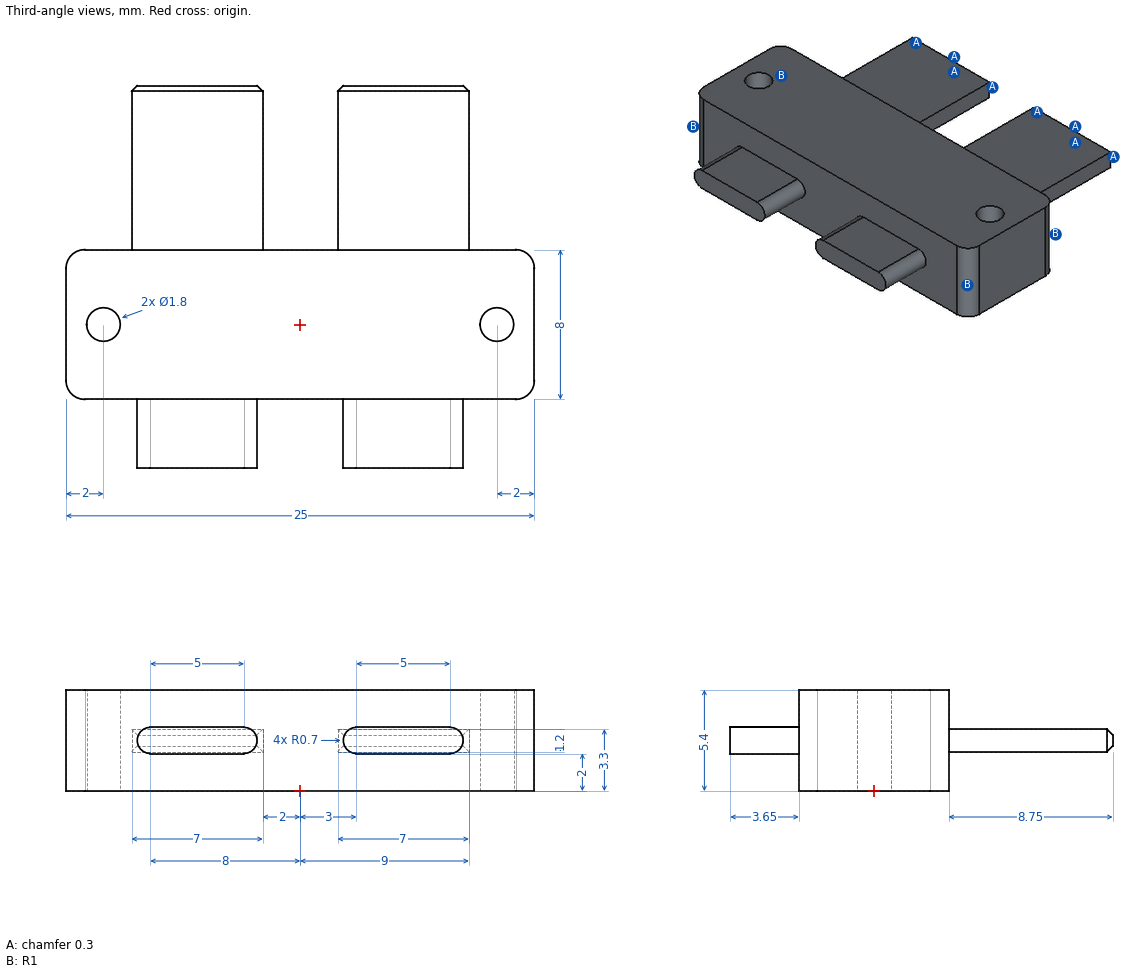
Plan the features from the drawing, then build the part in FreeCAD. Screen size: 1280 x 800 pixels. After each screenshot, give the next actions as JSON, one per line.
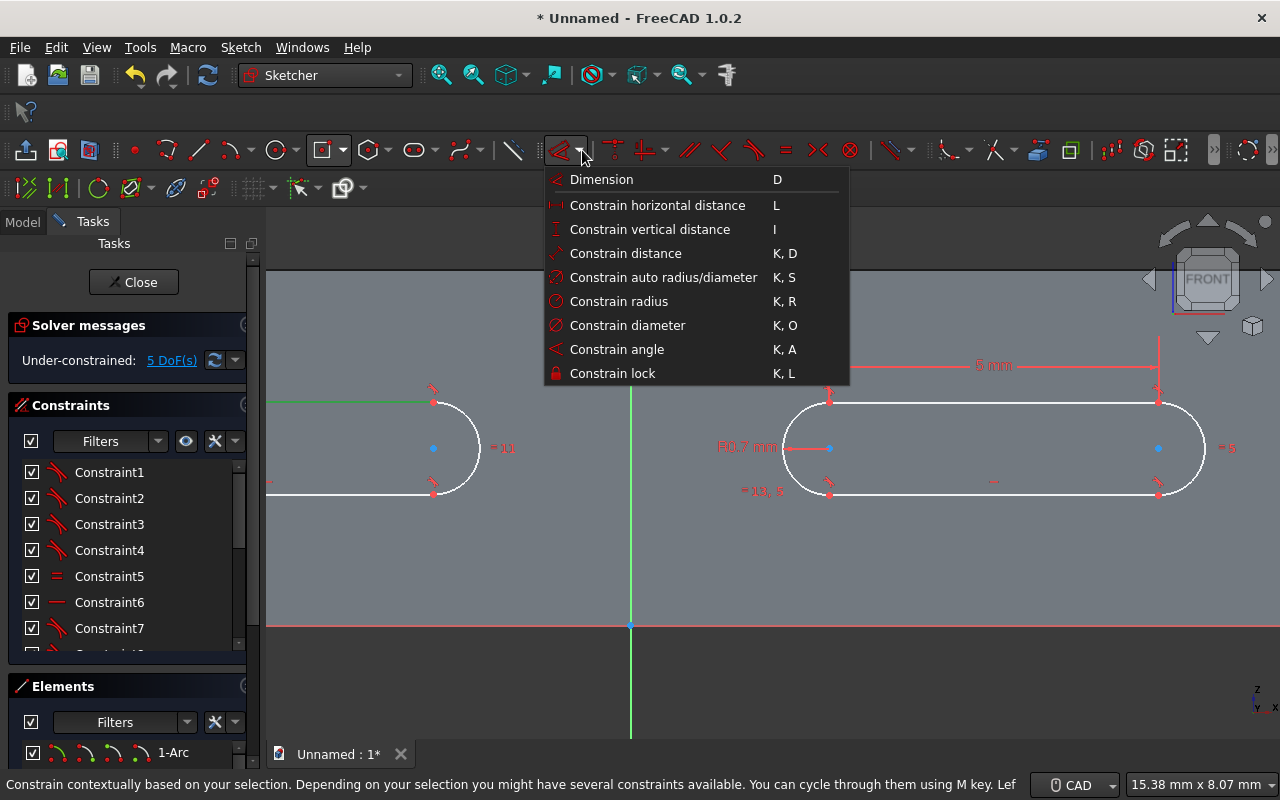
{"action": "left_click", "coordinate": [697, 205]}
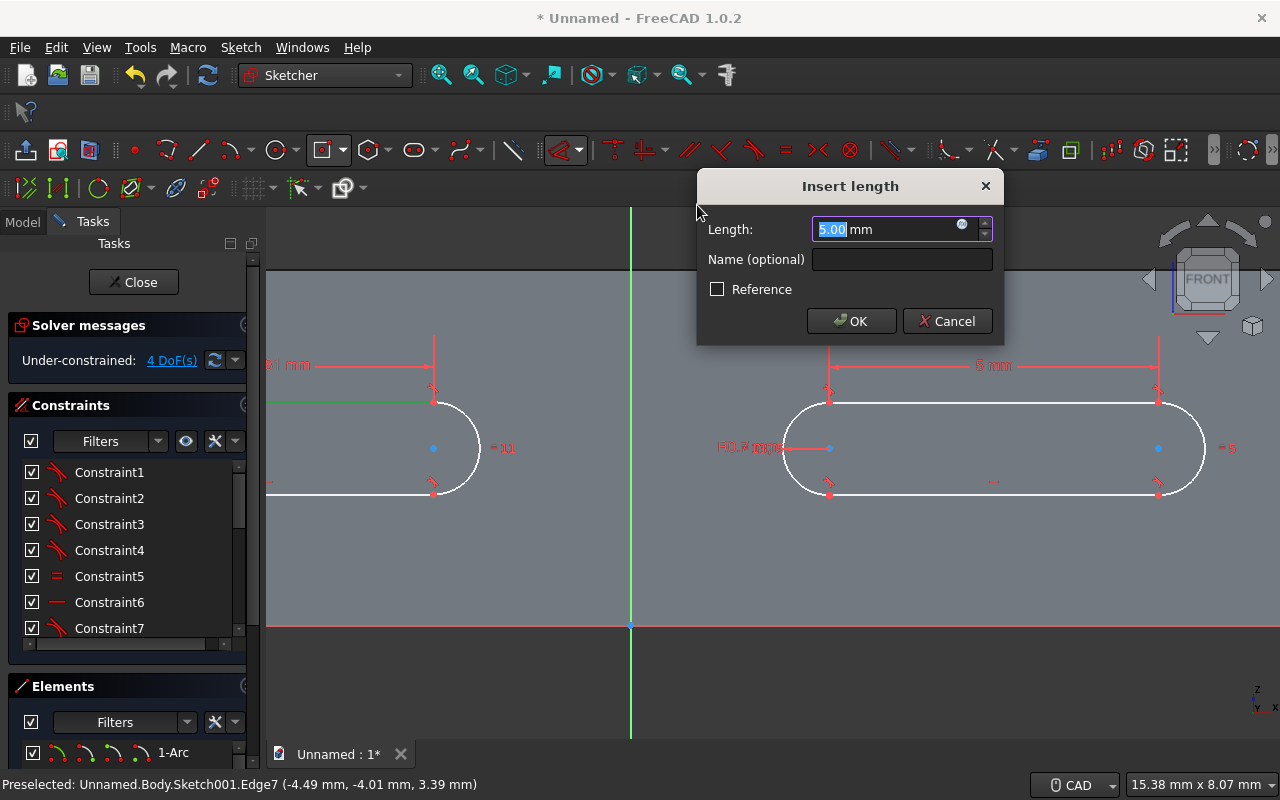
{"action": "type", "text": "5"}
{"action": "key", "text": "Return"}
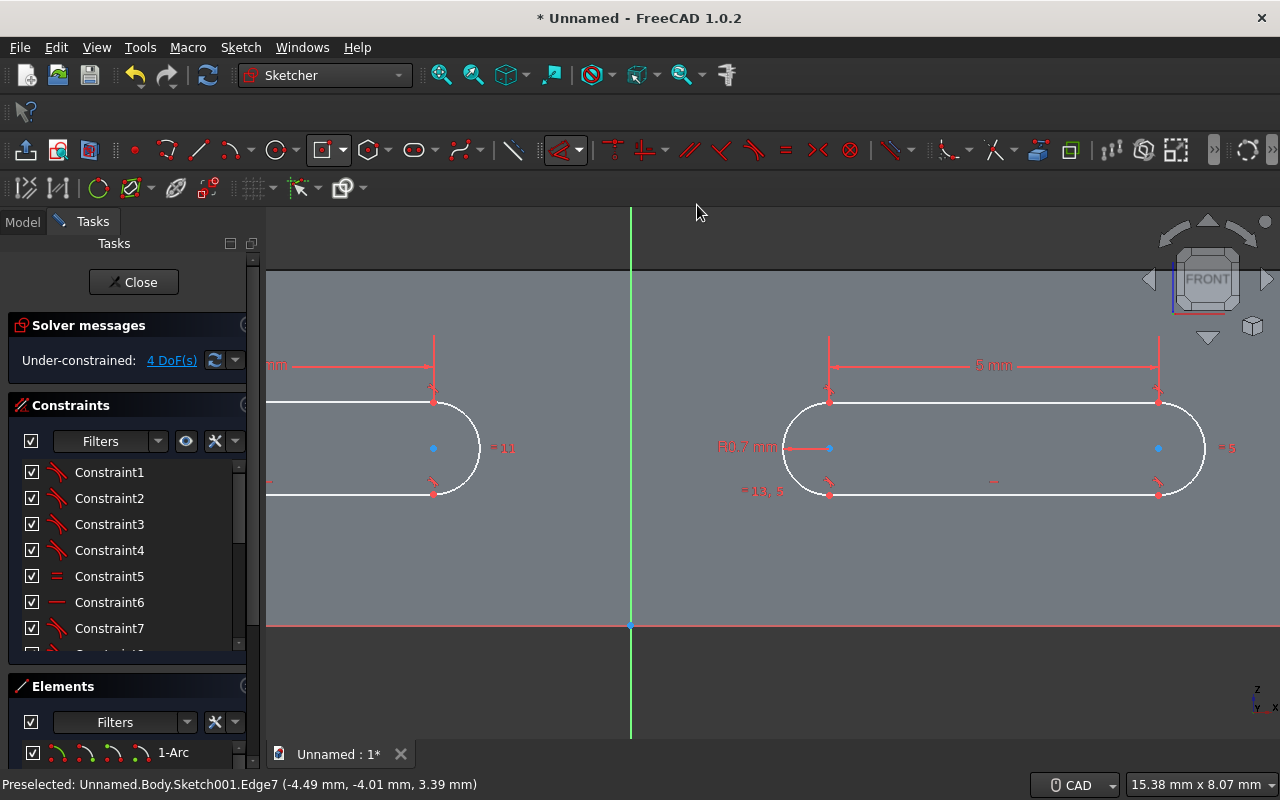
{"action": "left_click", "coordinate": [829, 403]}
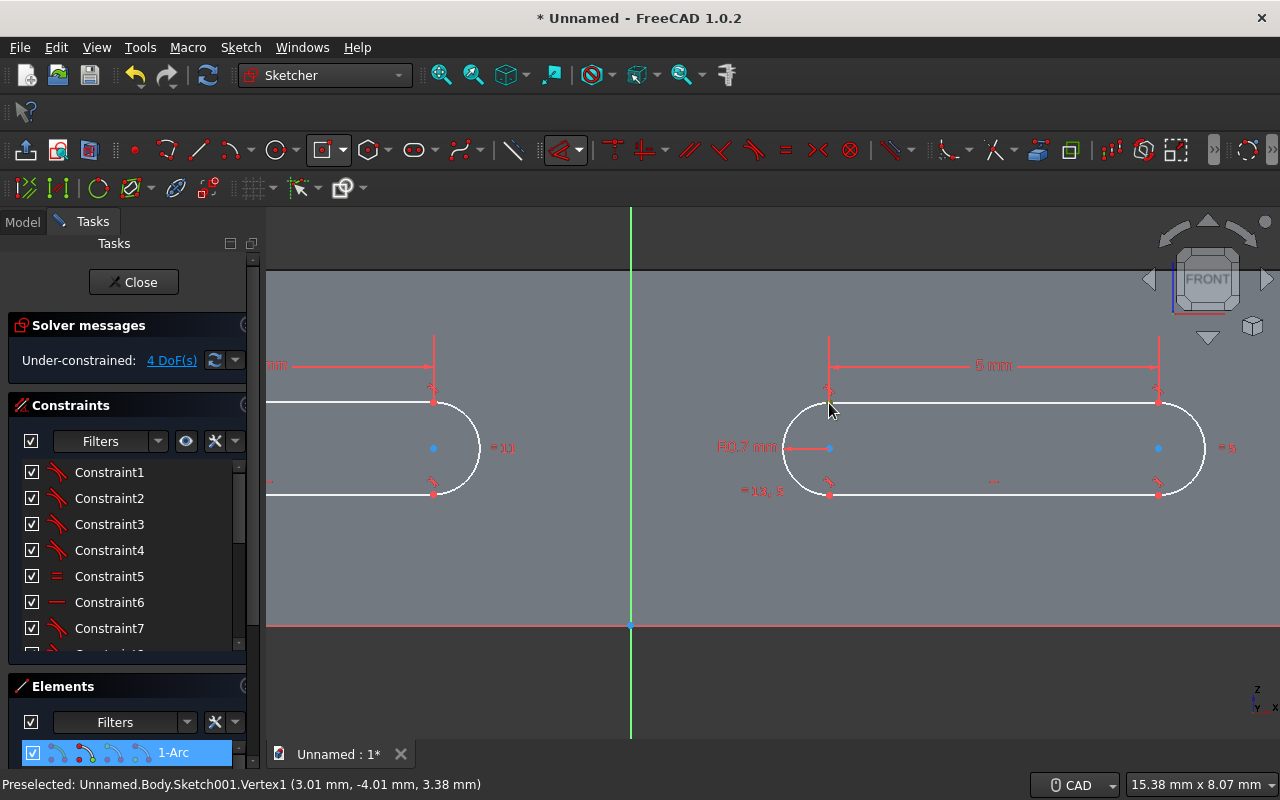
{"action": "key", "text": "l"}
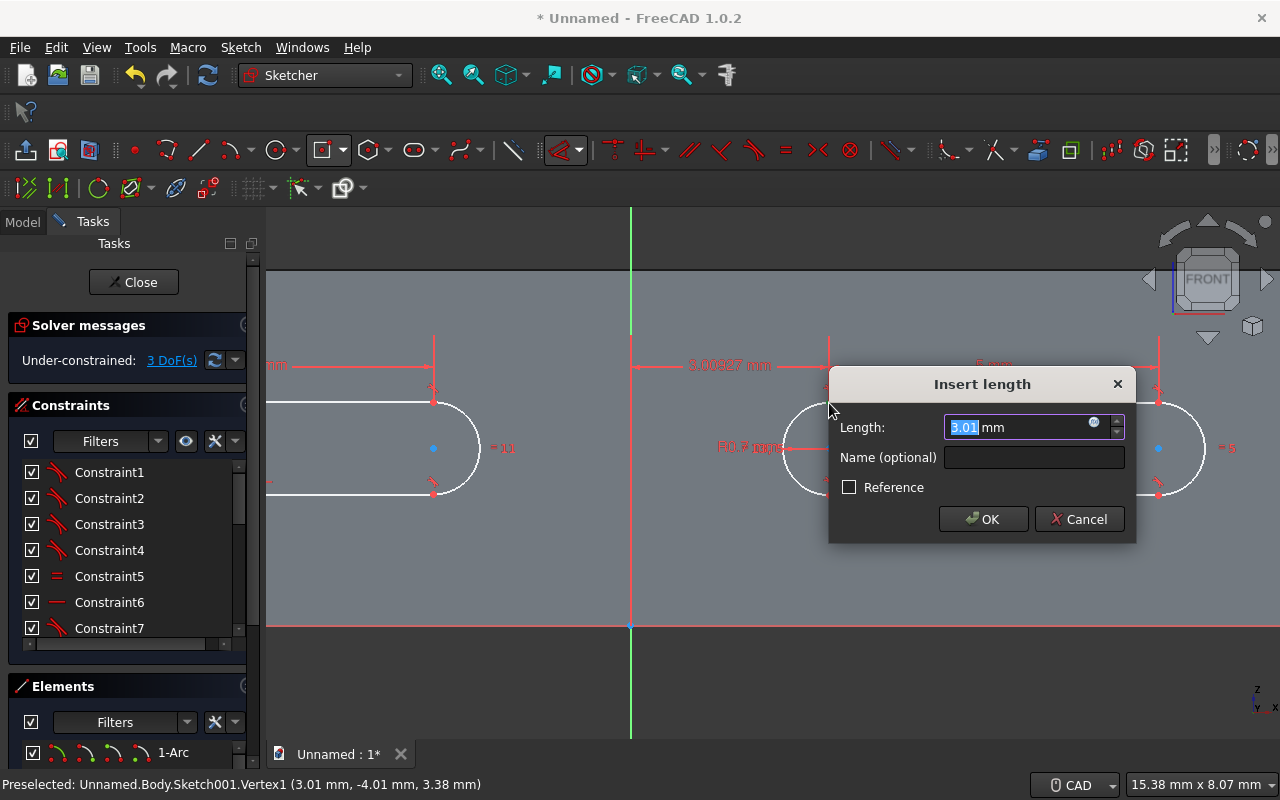
{"action": "type", "text": "3"}
{"action": "key", "text": "Return"}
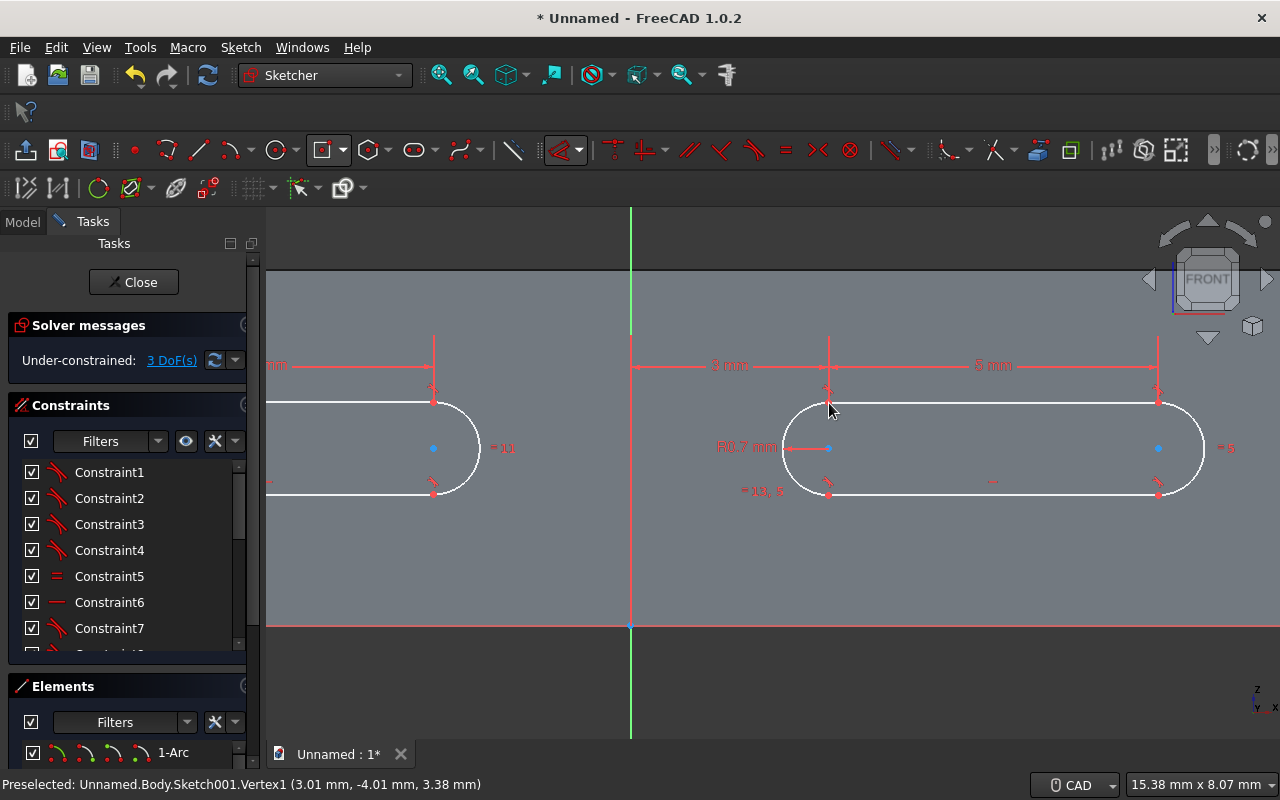
{"action": "left_click", "coordinate": [829, 495]}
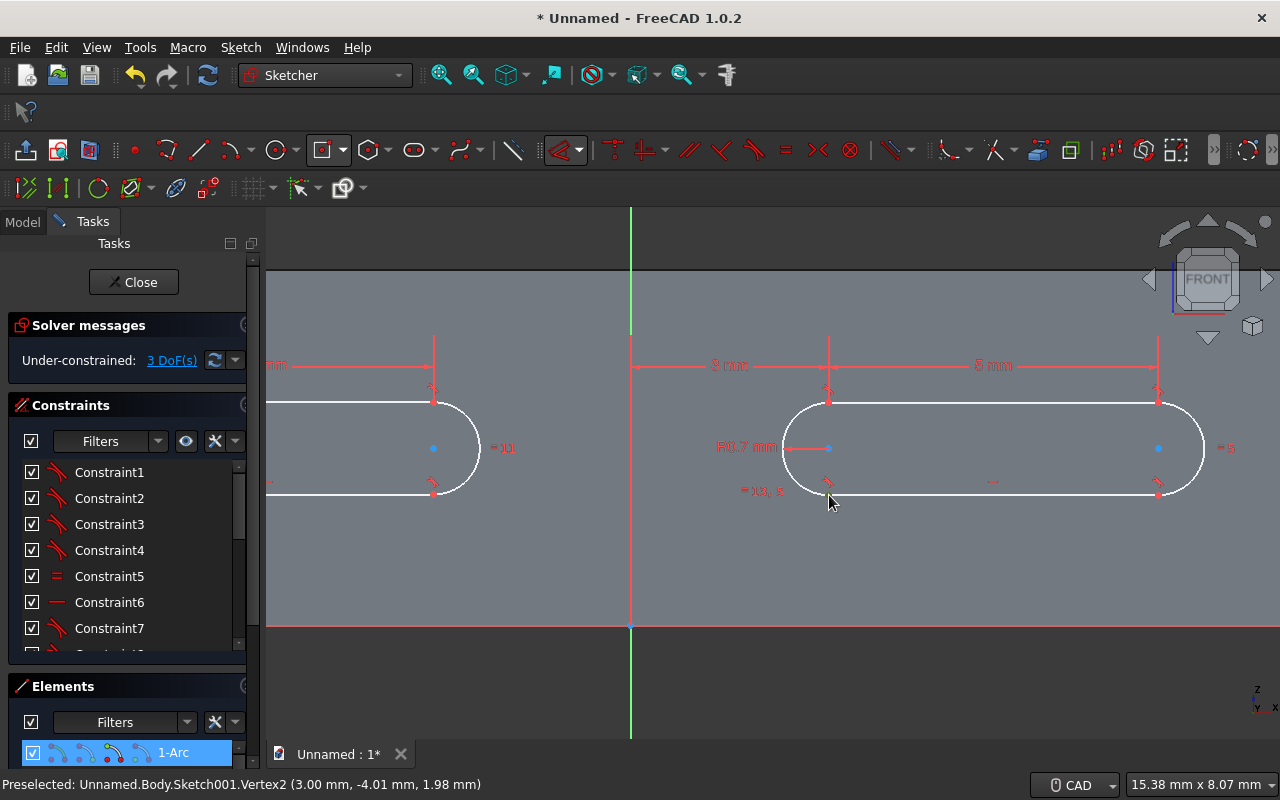
{"action": "left_click", "coordinate": [582, 150]}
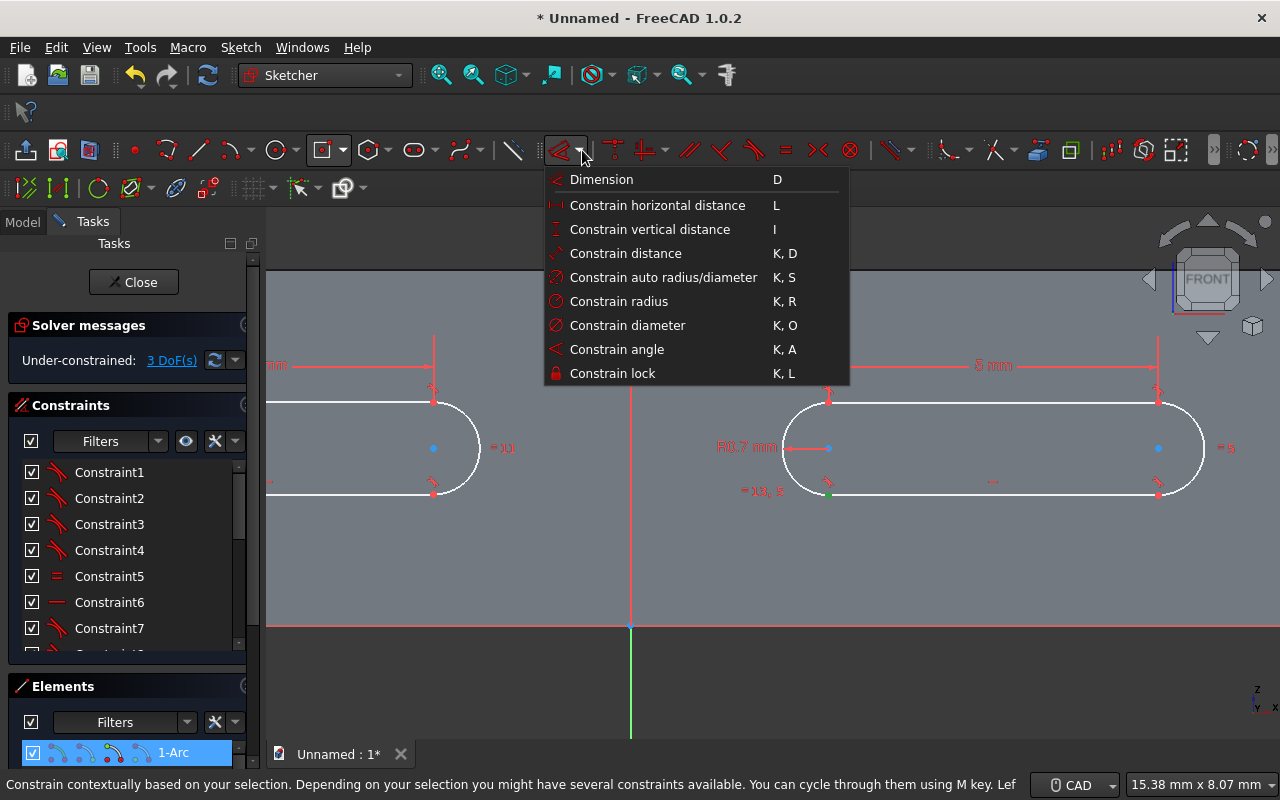
{"action": "left_click", "coordinate": [697, 229]}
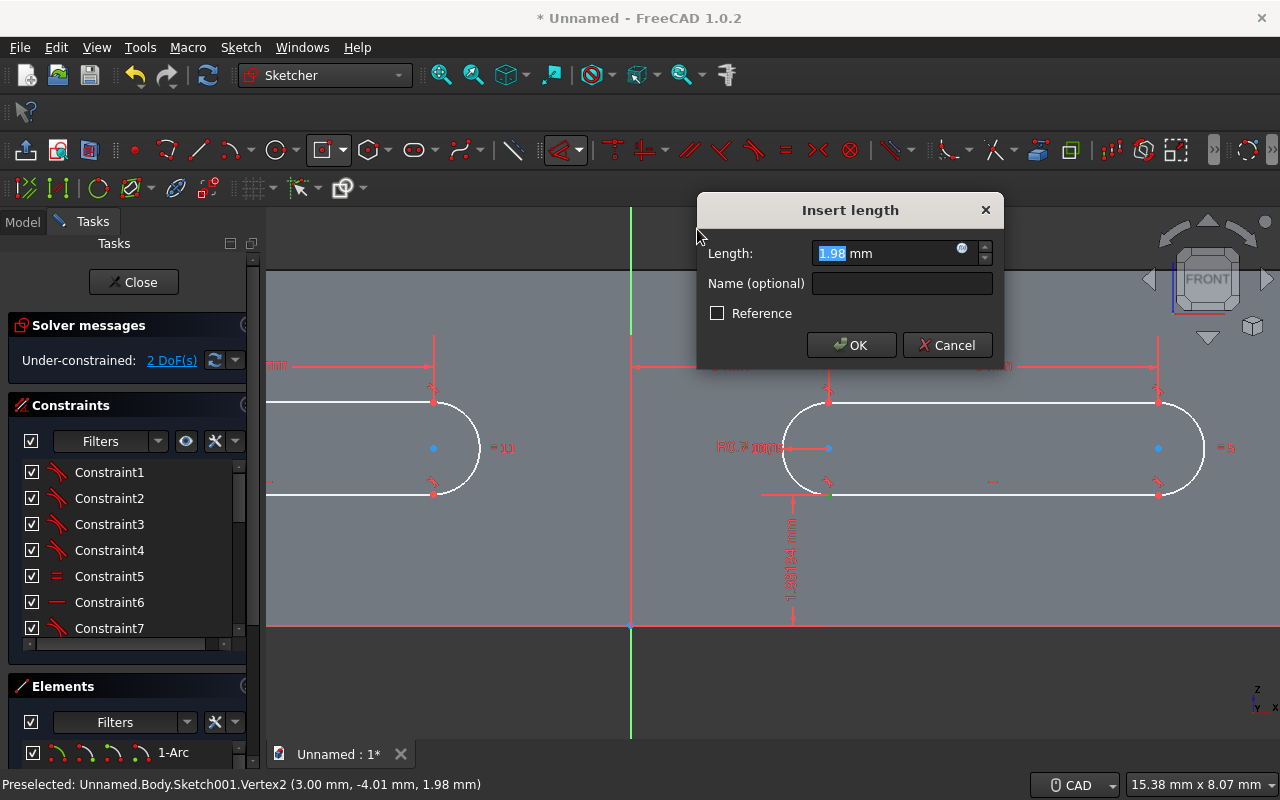
{"action": "type", "text": "2"}
{"action": "key", "text": "Return"}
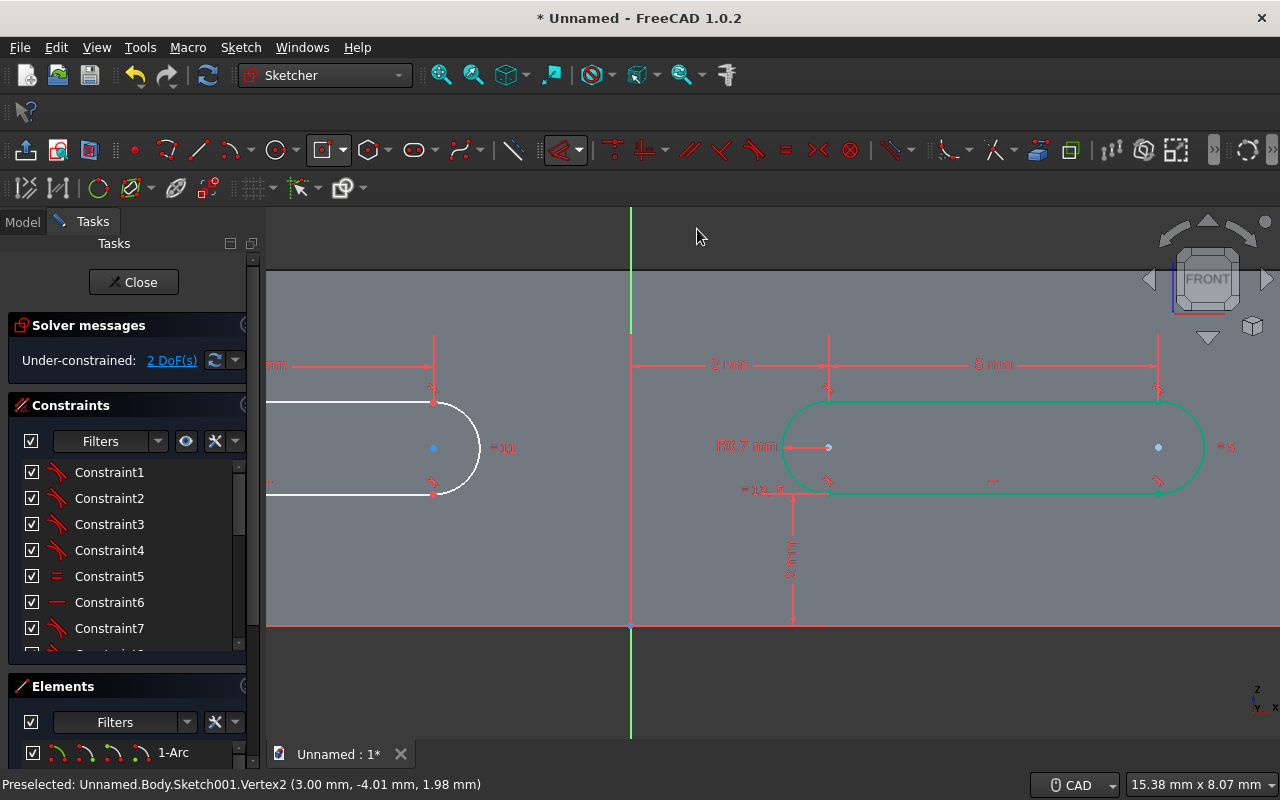
{"action": "scroll", "coordinate": [794, 423], "scroll_direction": "down", "scroll_amount": 3}